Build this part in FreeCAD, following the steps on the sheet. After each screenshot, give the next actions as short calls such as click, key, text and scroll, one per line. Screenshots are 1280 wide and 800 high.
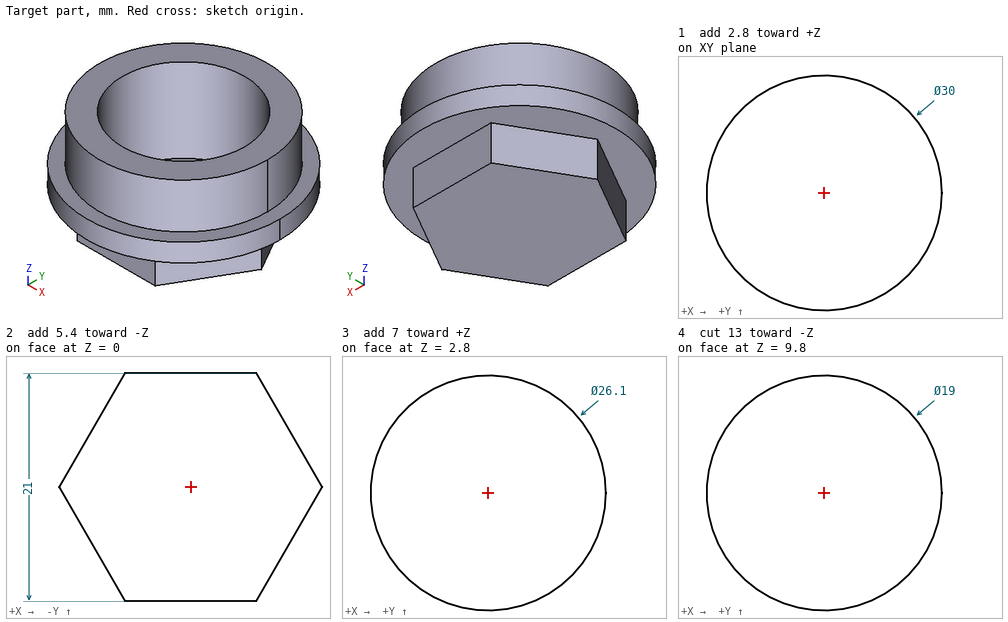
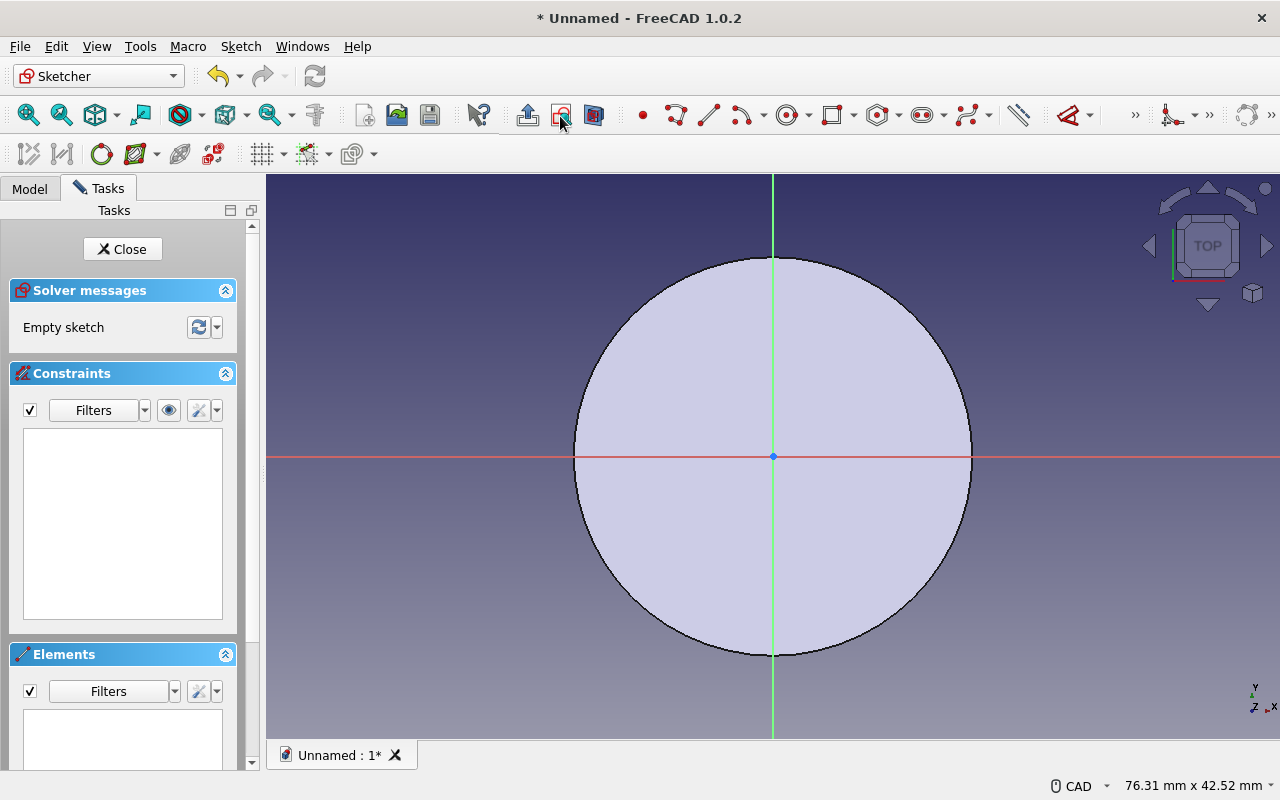
click(786, 116)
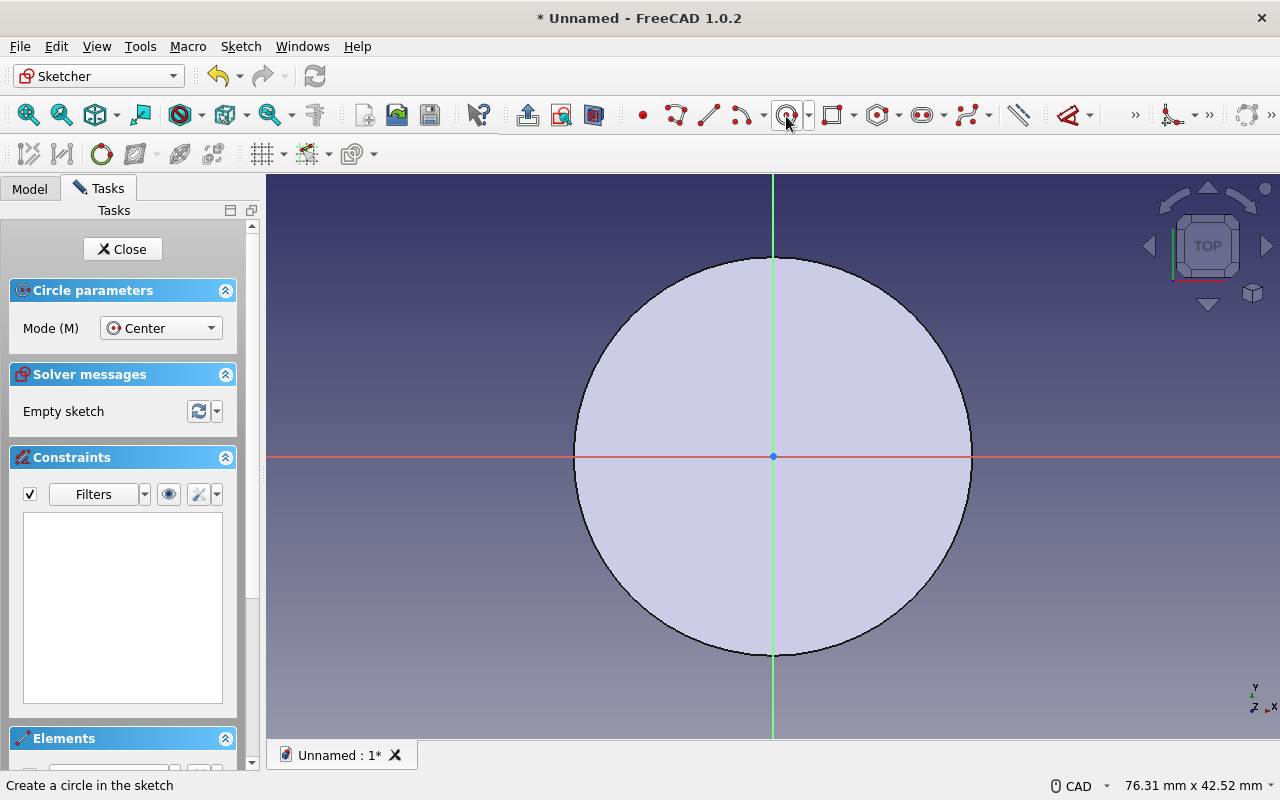
click(773, 456)
move(896, 334)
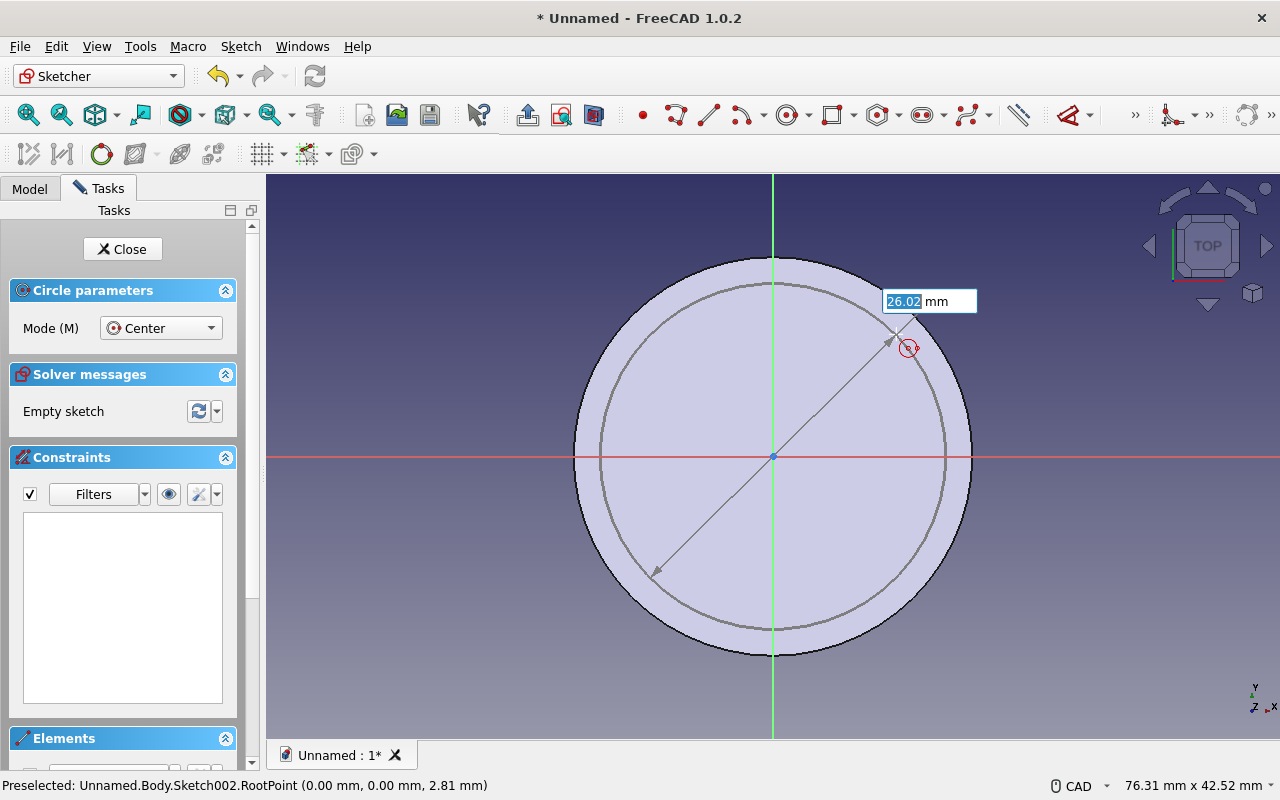
text(26.1)
key(Return)
key(Escape)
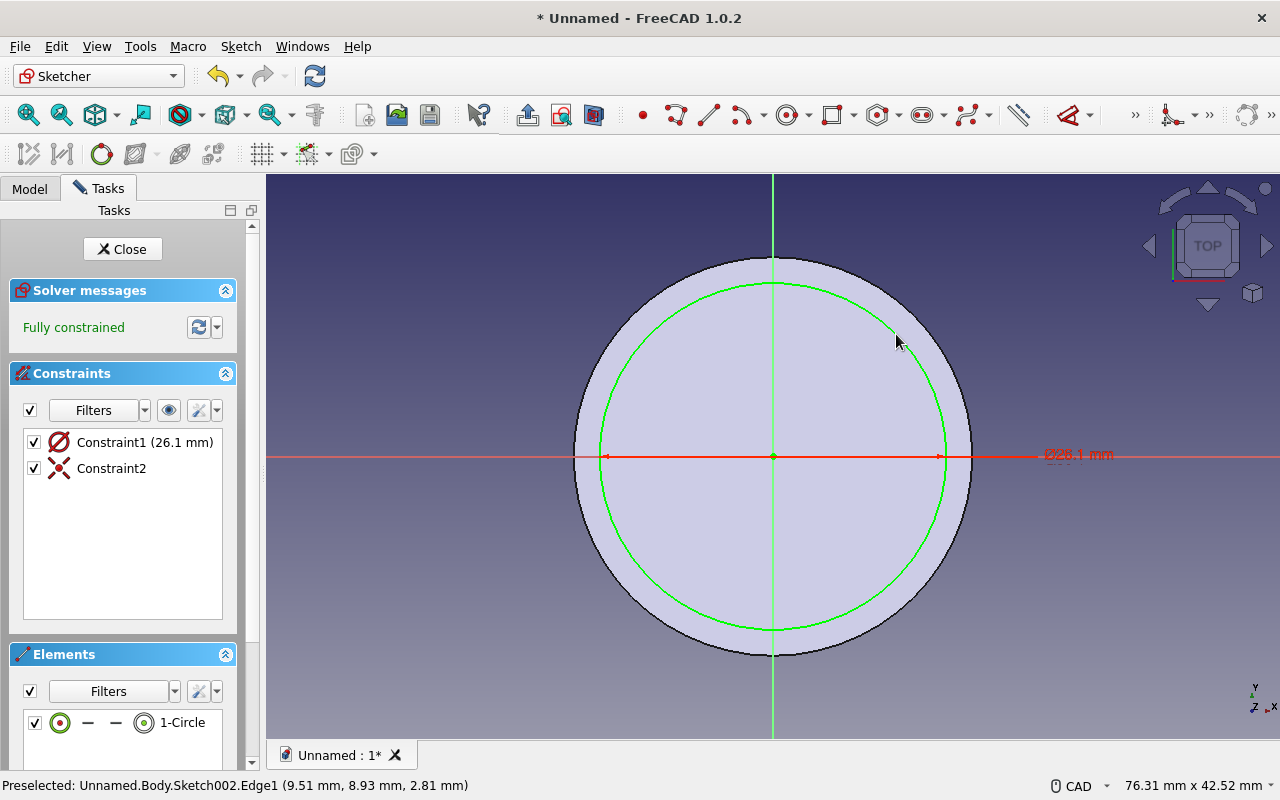
click(123, 249)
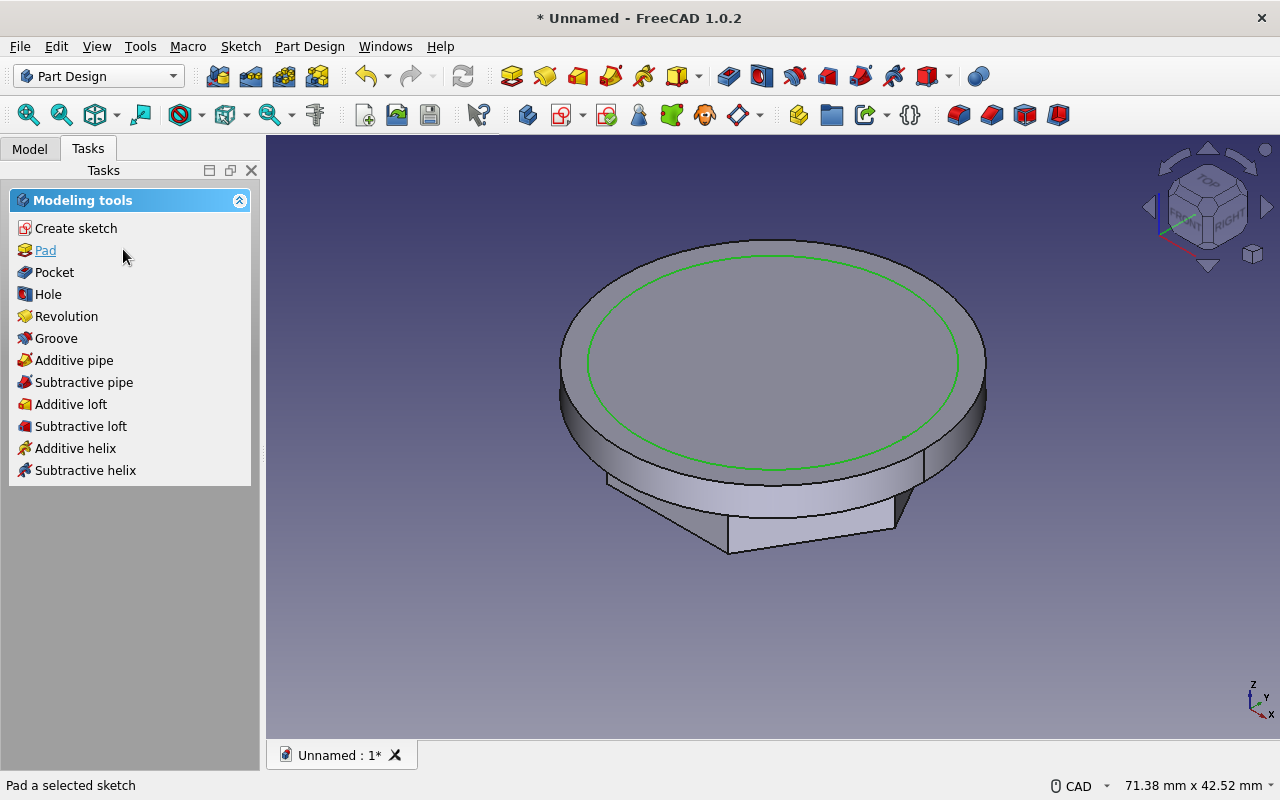
click(512, 76)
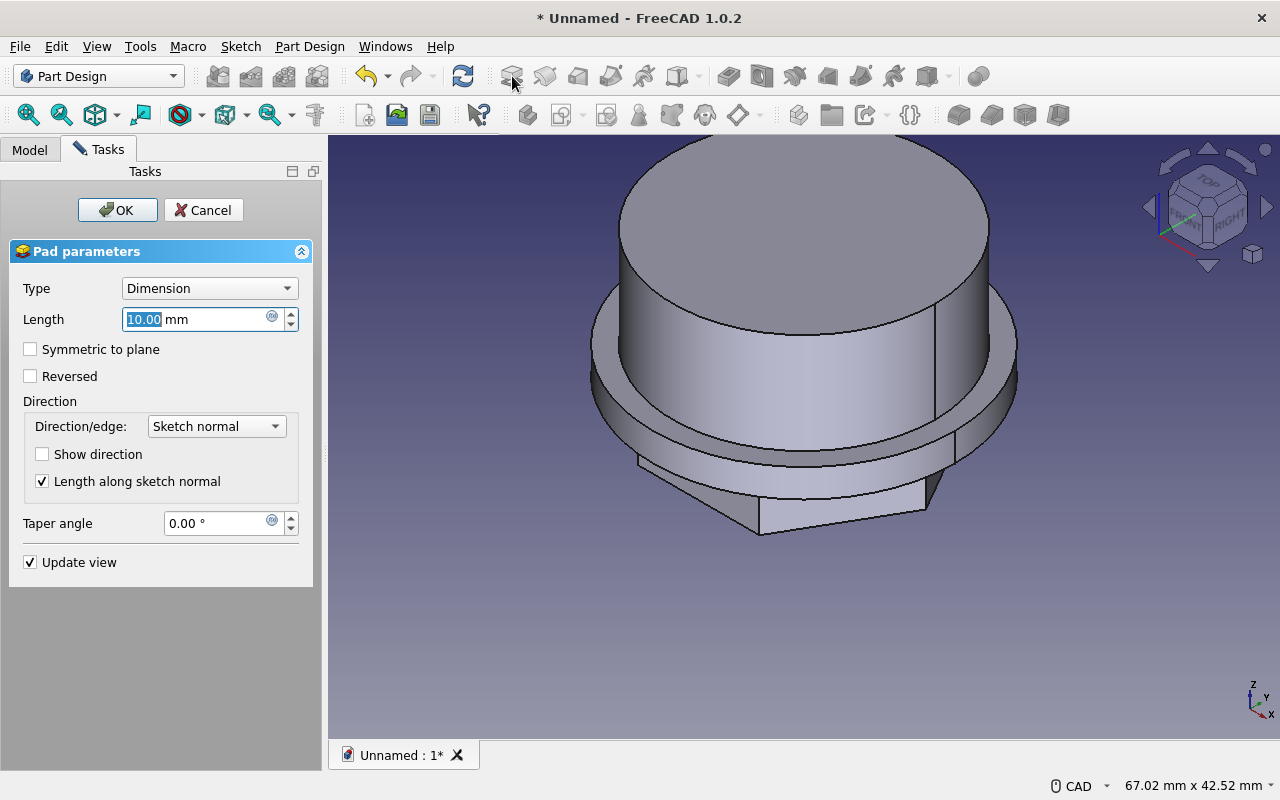
text(7)
key(Tab)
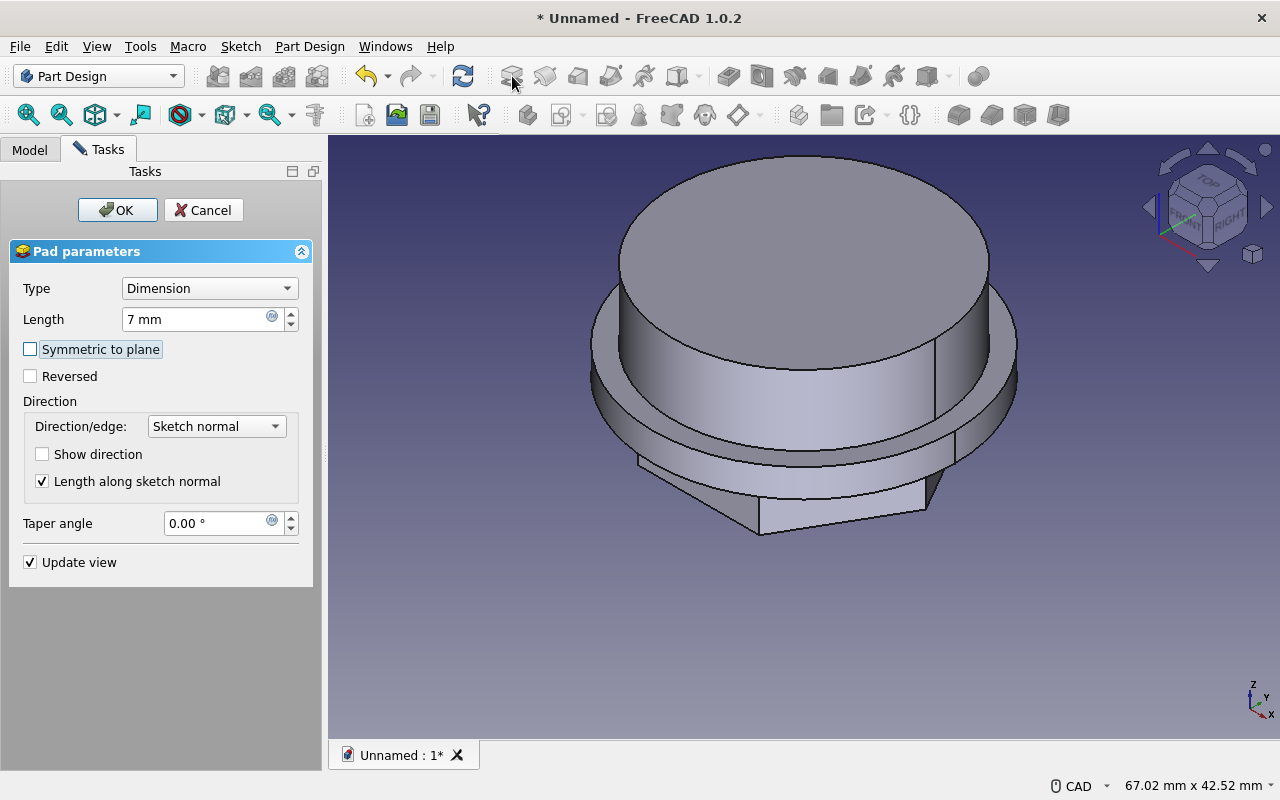
click(118, 210)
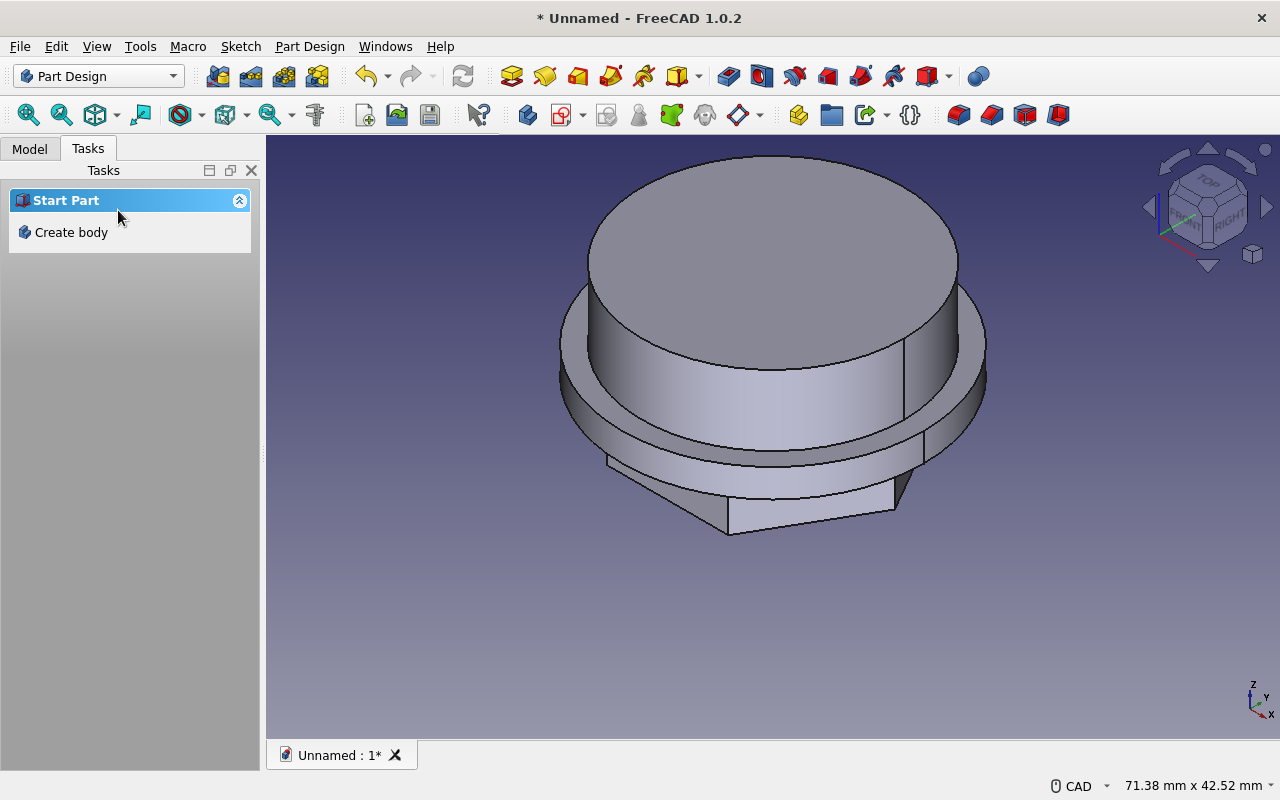
click(29, 116)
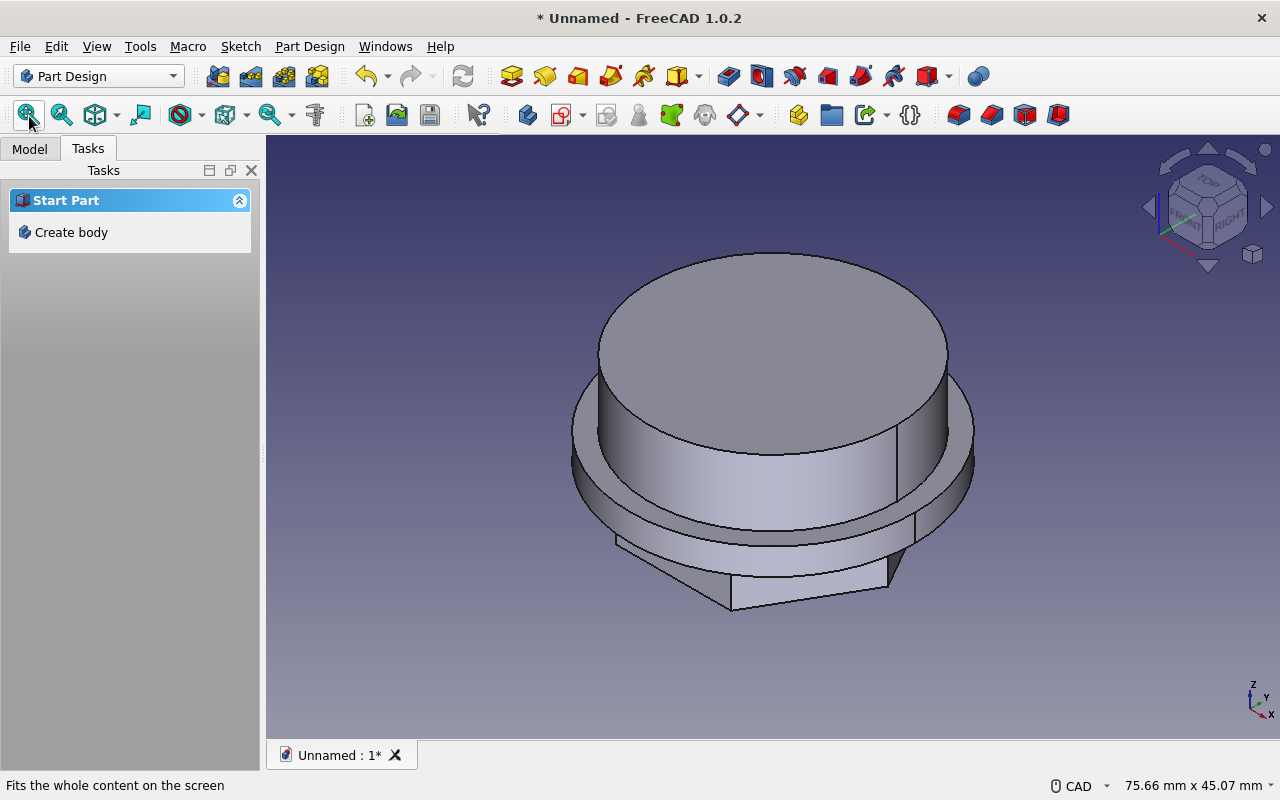
click(773, 353)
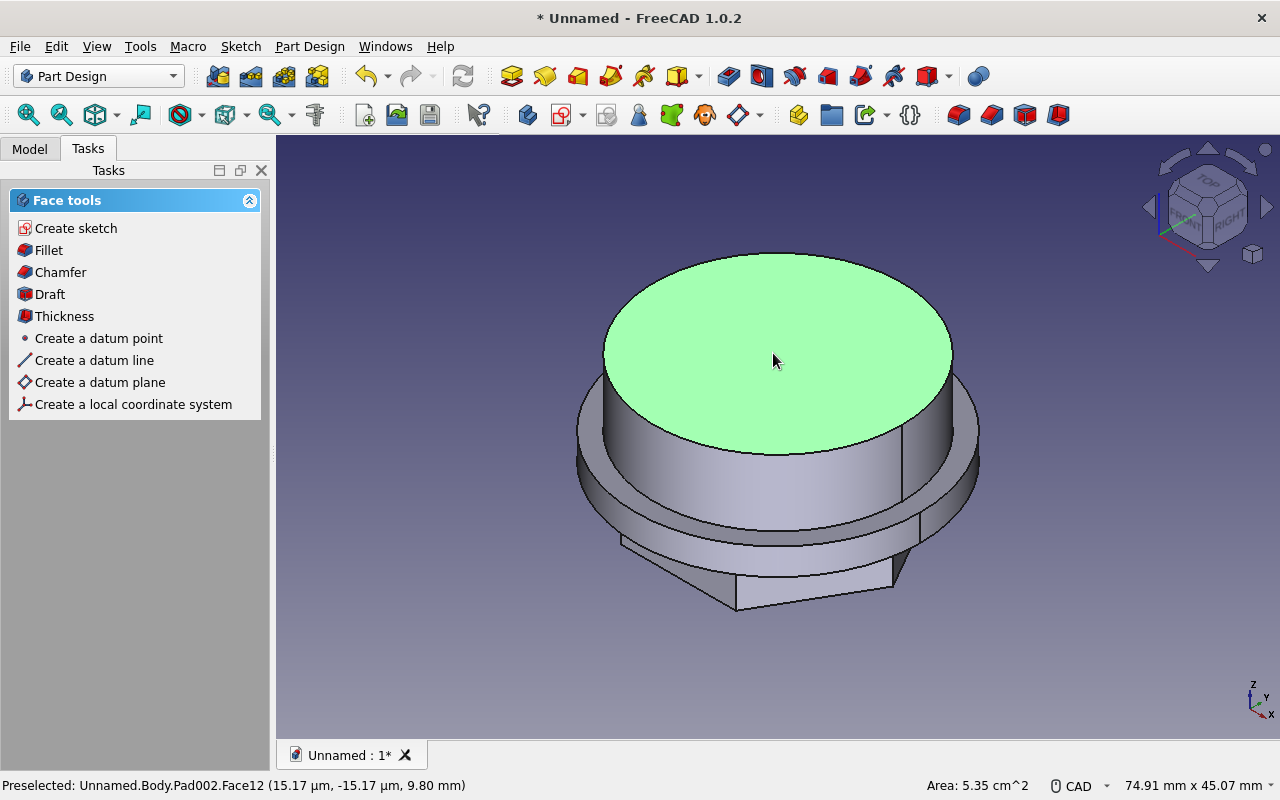
click(560, 116)